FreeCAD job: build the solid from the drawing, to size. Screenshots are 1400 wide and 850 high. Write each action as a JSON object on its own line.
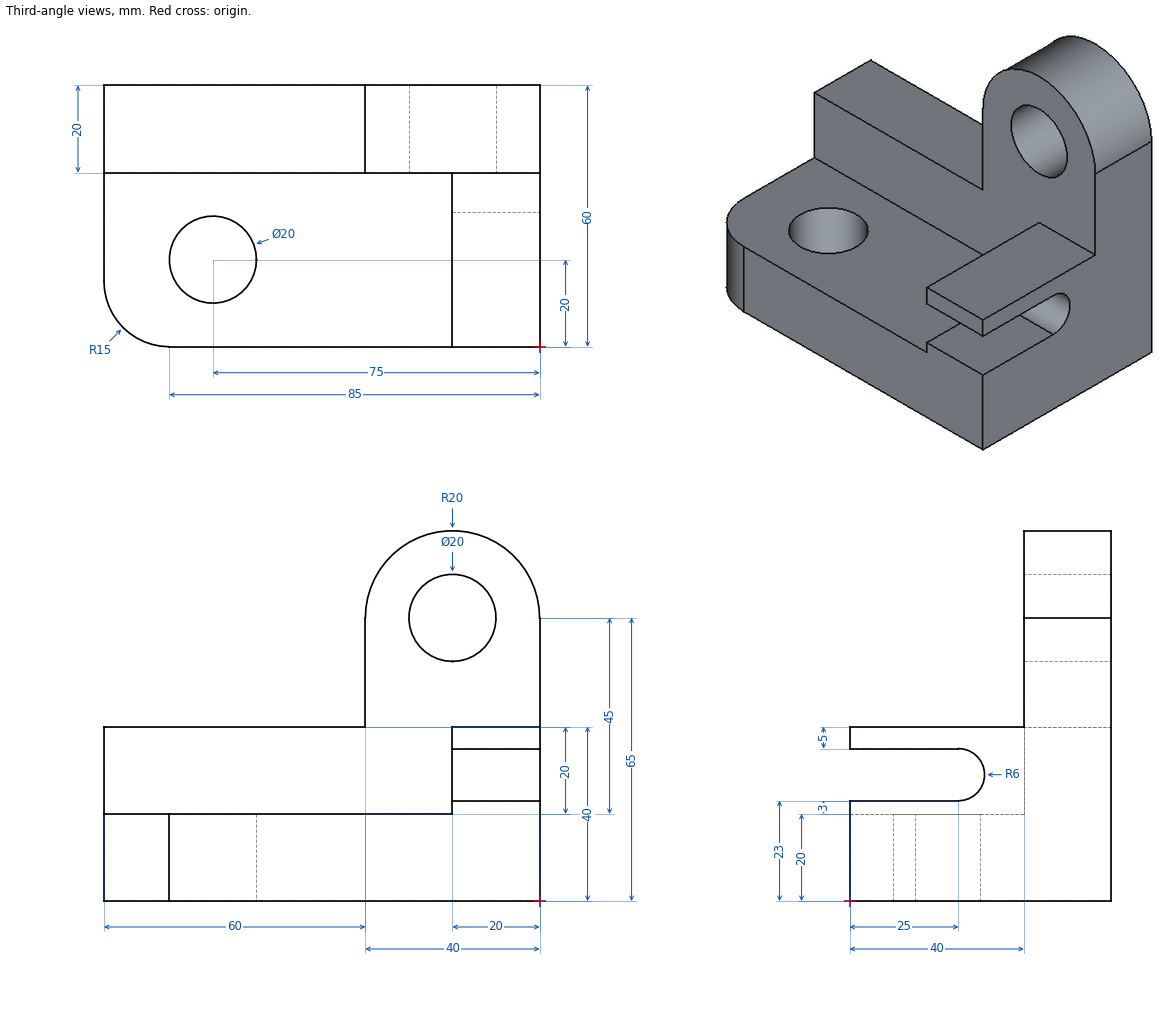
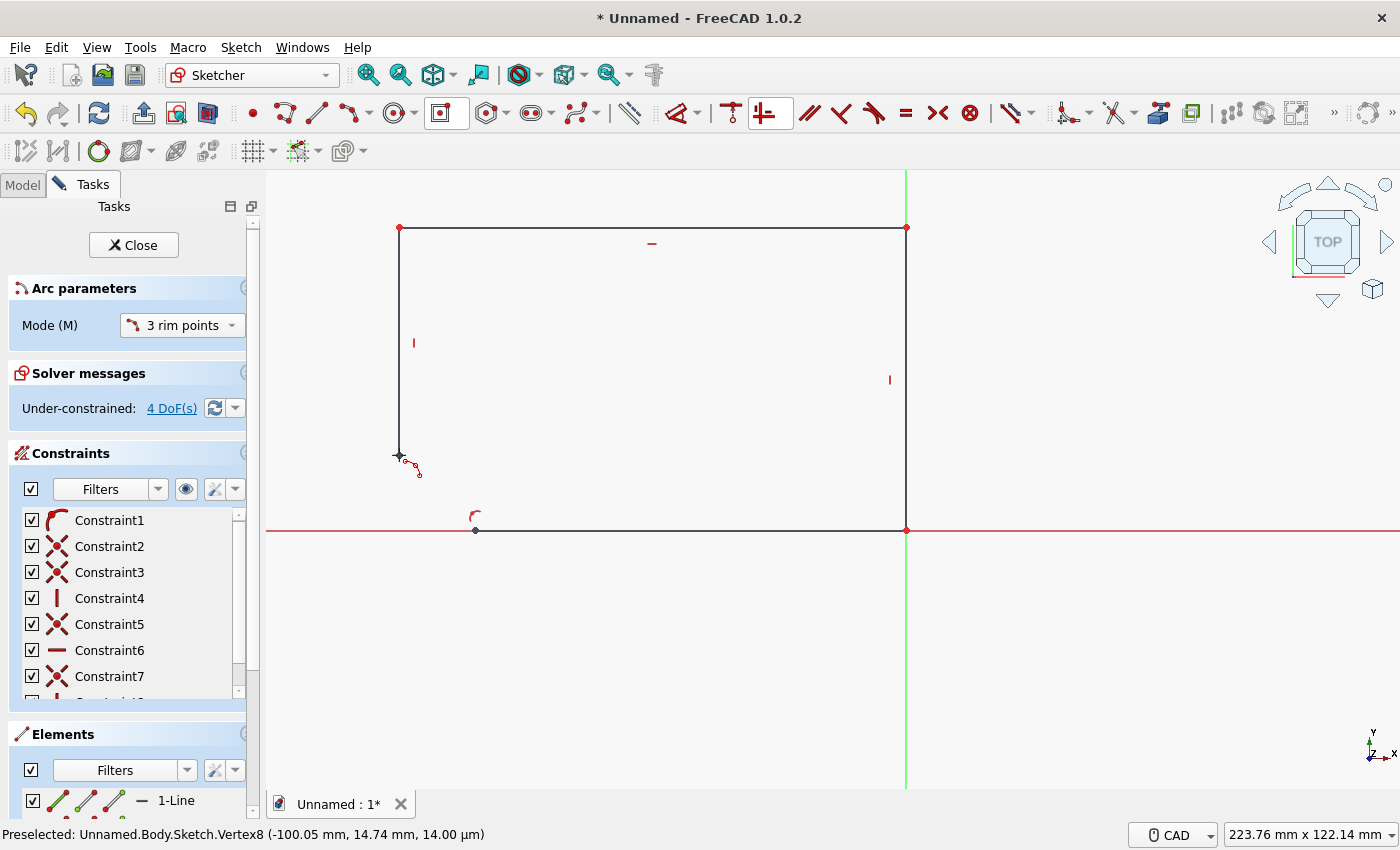
{"action": "left_click", "coordinate": [399, 456]}
{"action": "left_click", "coordinate": [475, 531]}
{"action": "left_click", "coordinate": [421, 508]}
{"action": "key", "text": "Escape"}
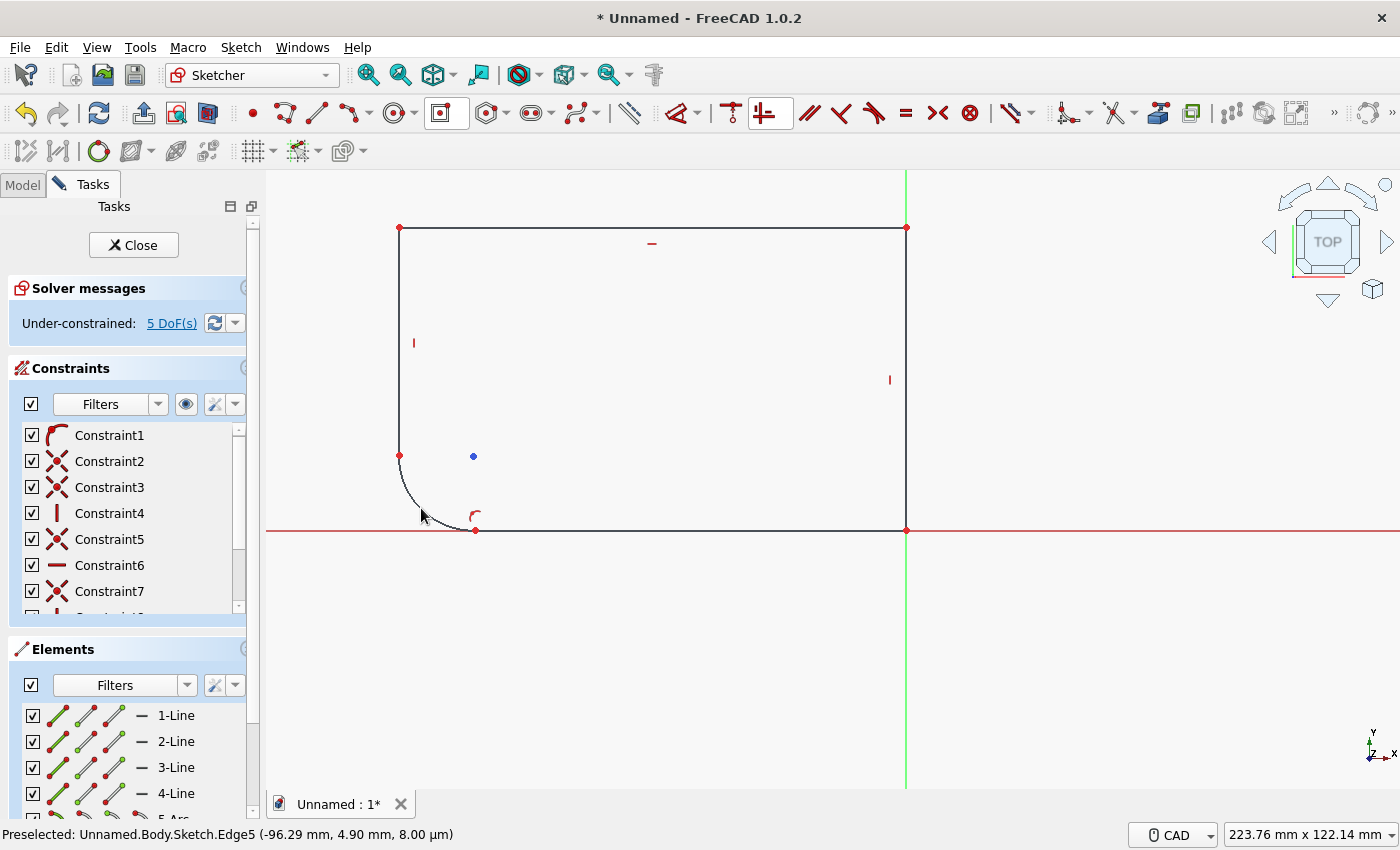
{"action": "left_click", "coordinate": [604, 531]}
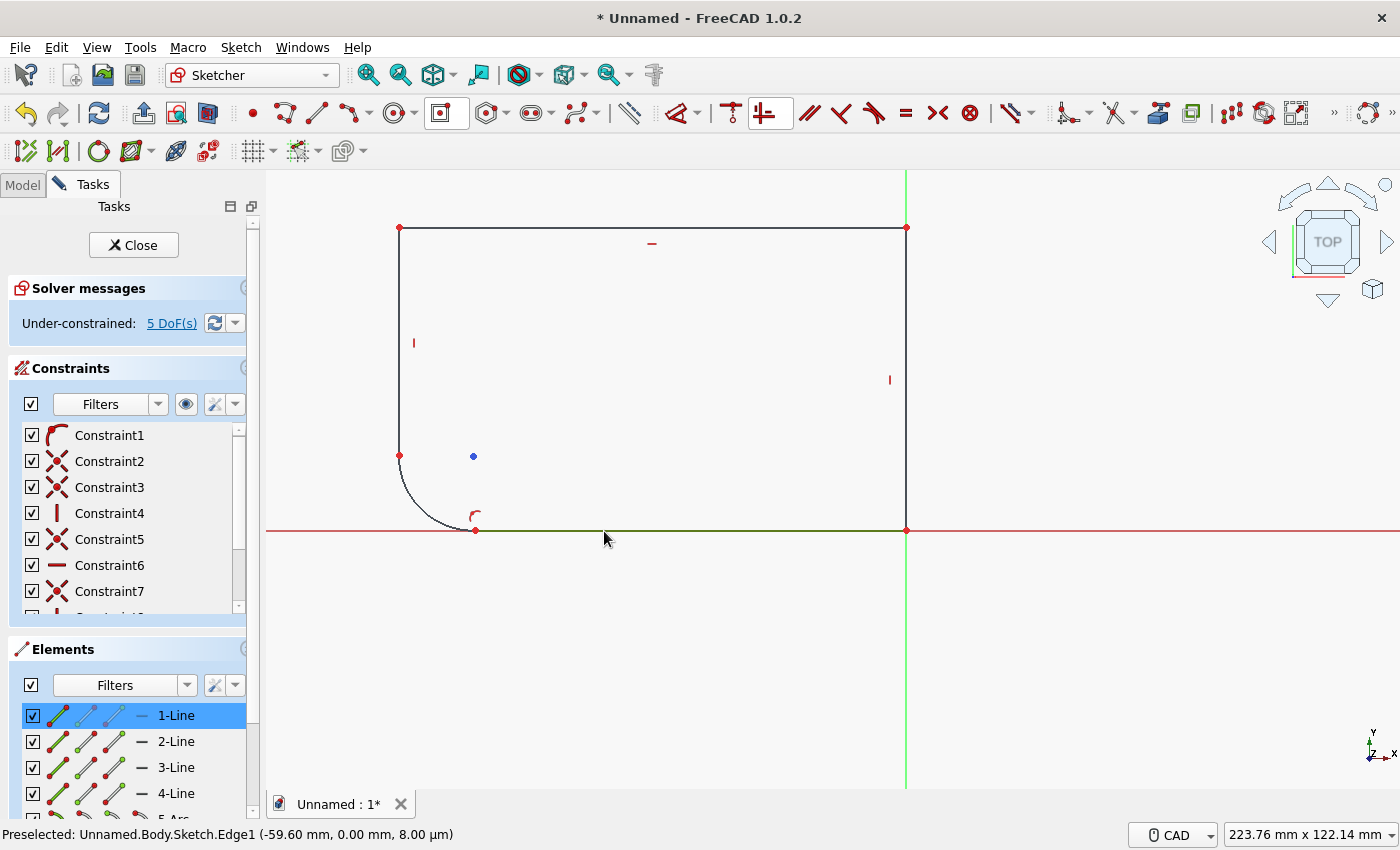
{"action": "left_click", "coordinate": [407, 490]}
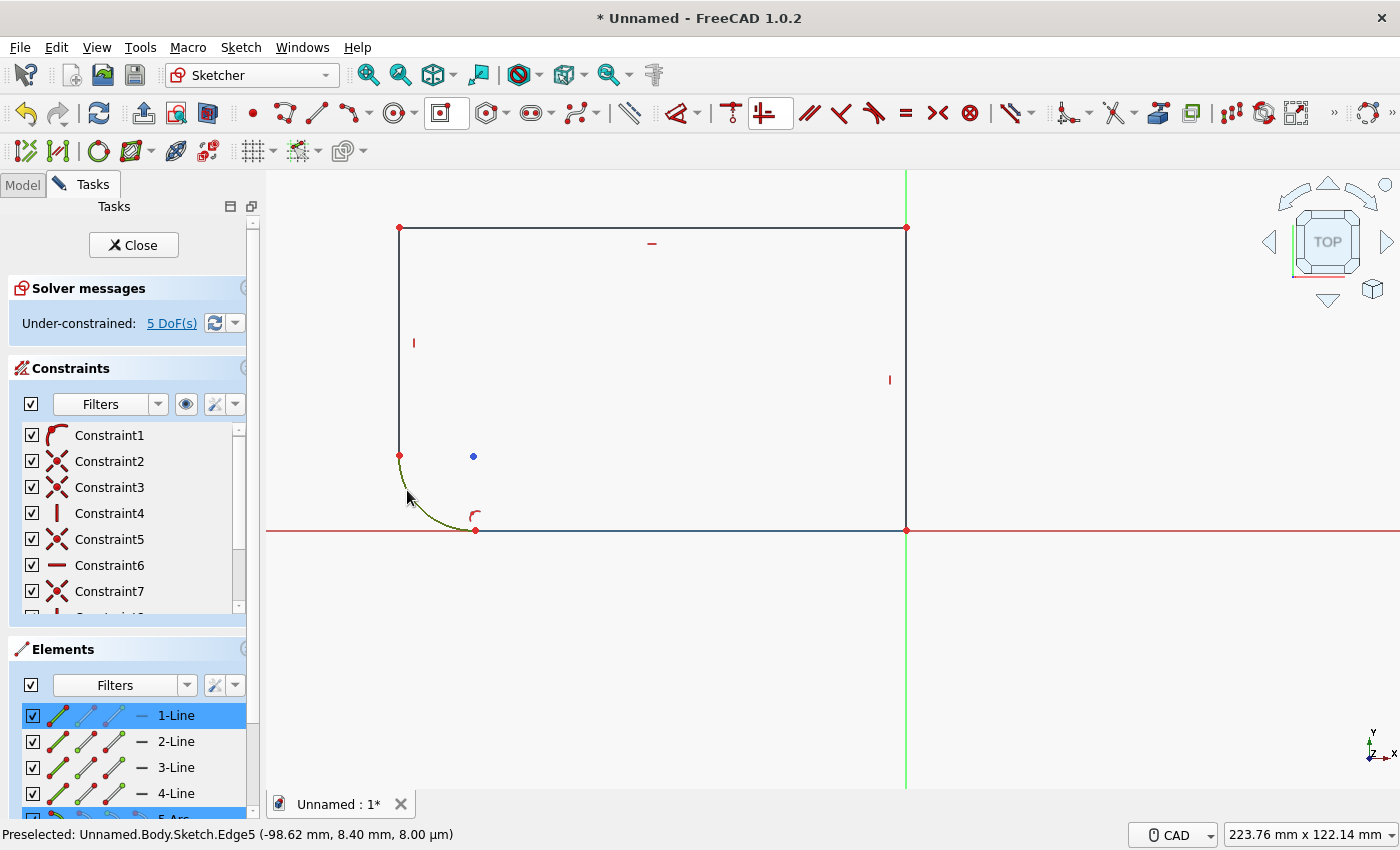
{"action": "left_click", "coordinate": [874, 114]}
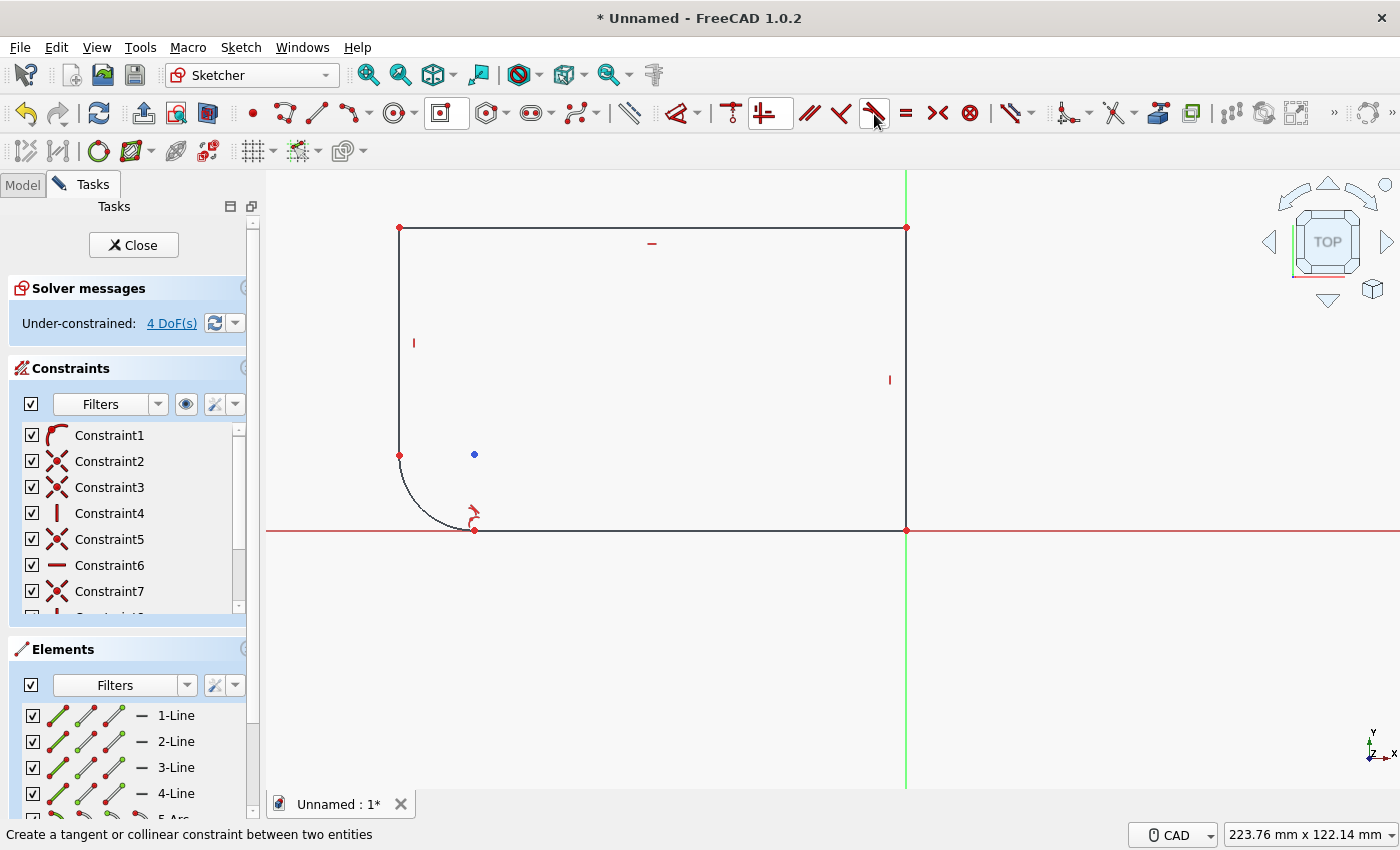
{"action": "left_click", "coordinate": [399, 296]}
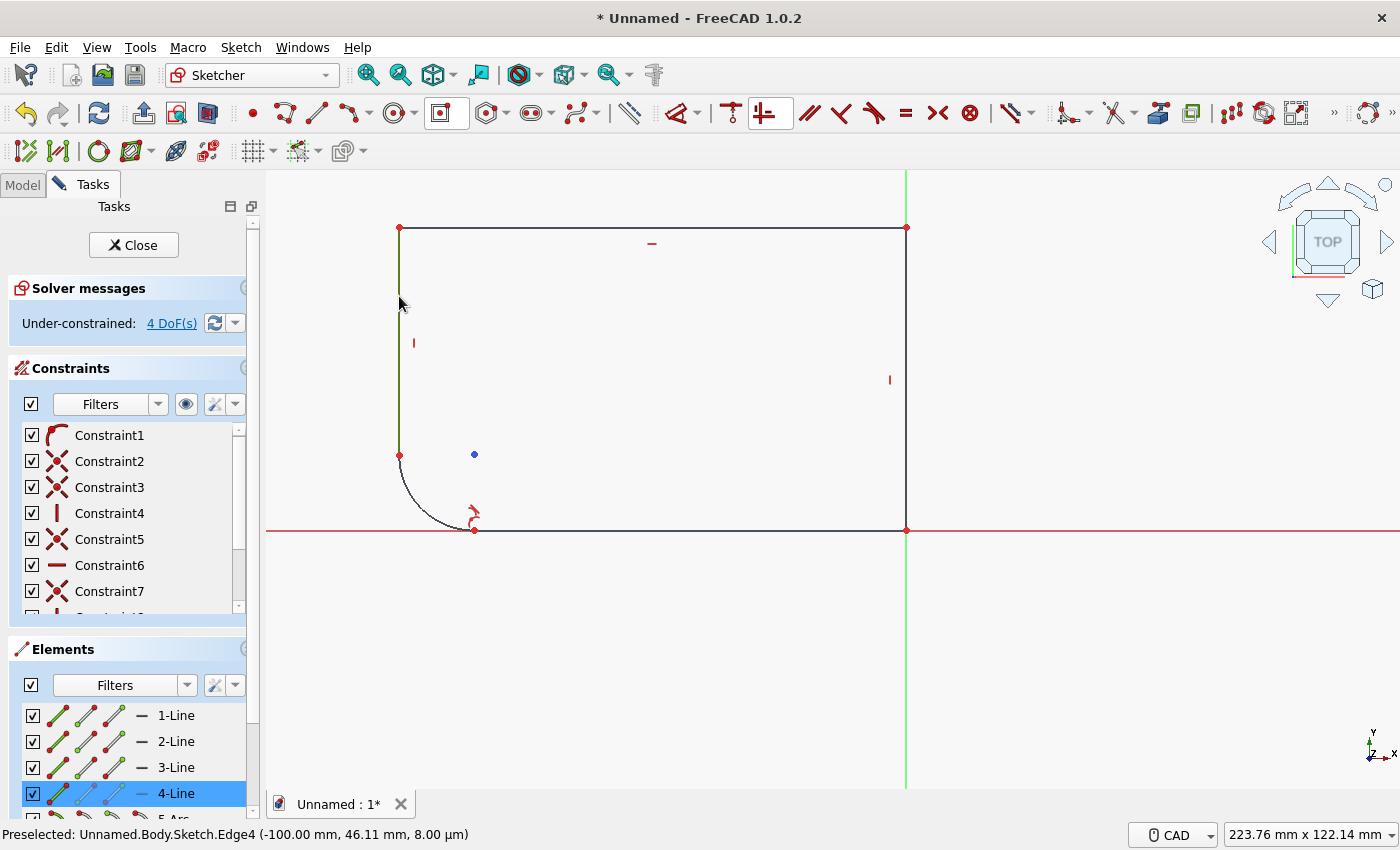
{"action": "left_click", "coordinate": [408, 490]}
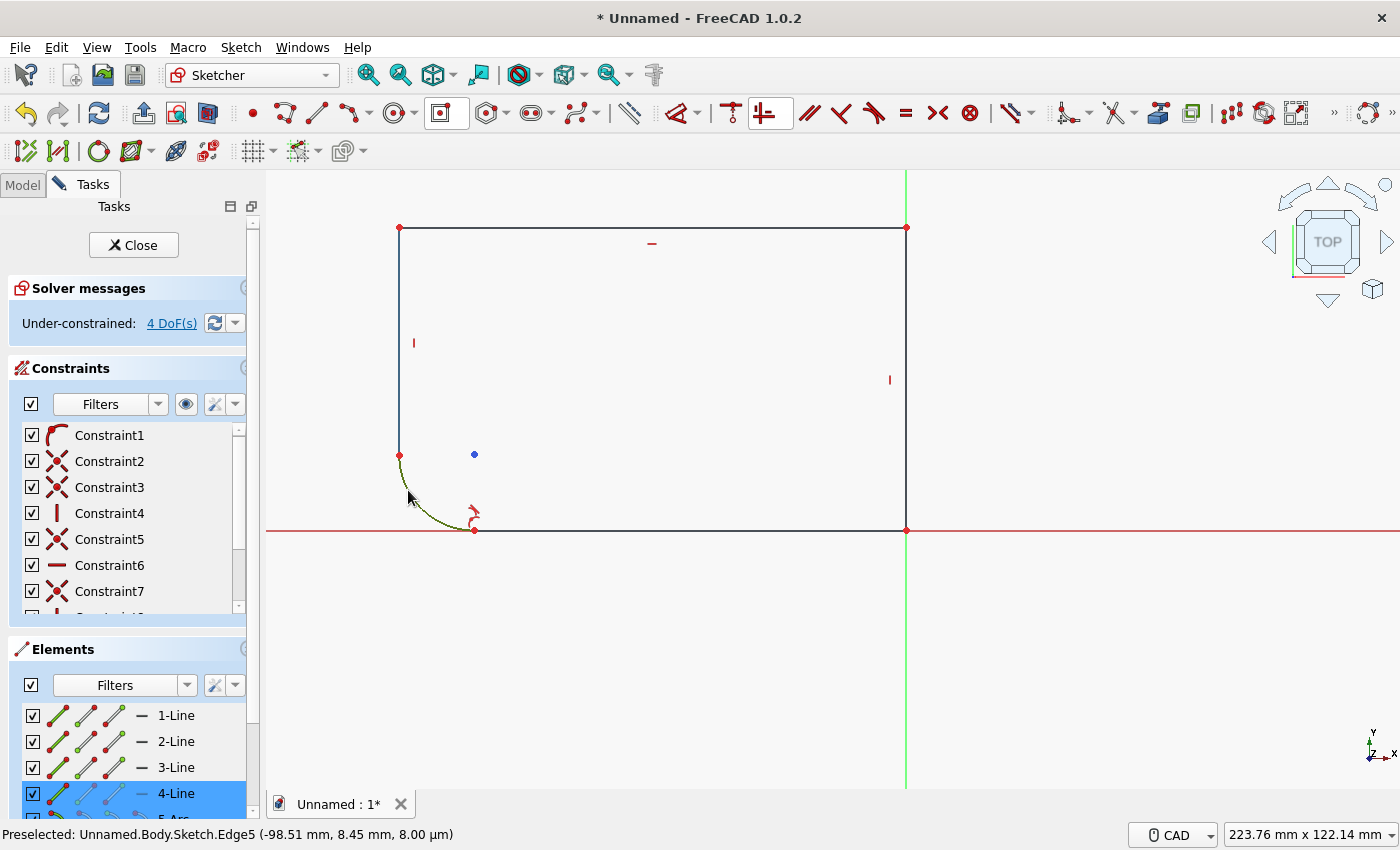
{"action": "key", "text": "t"}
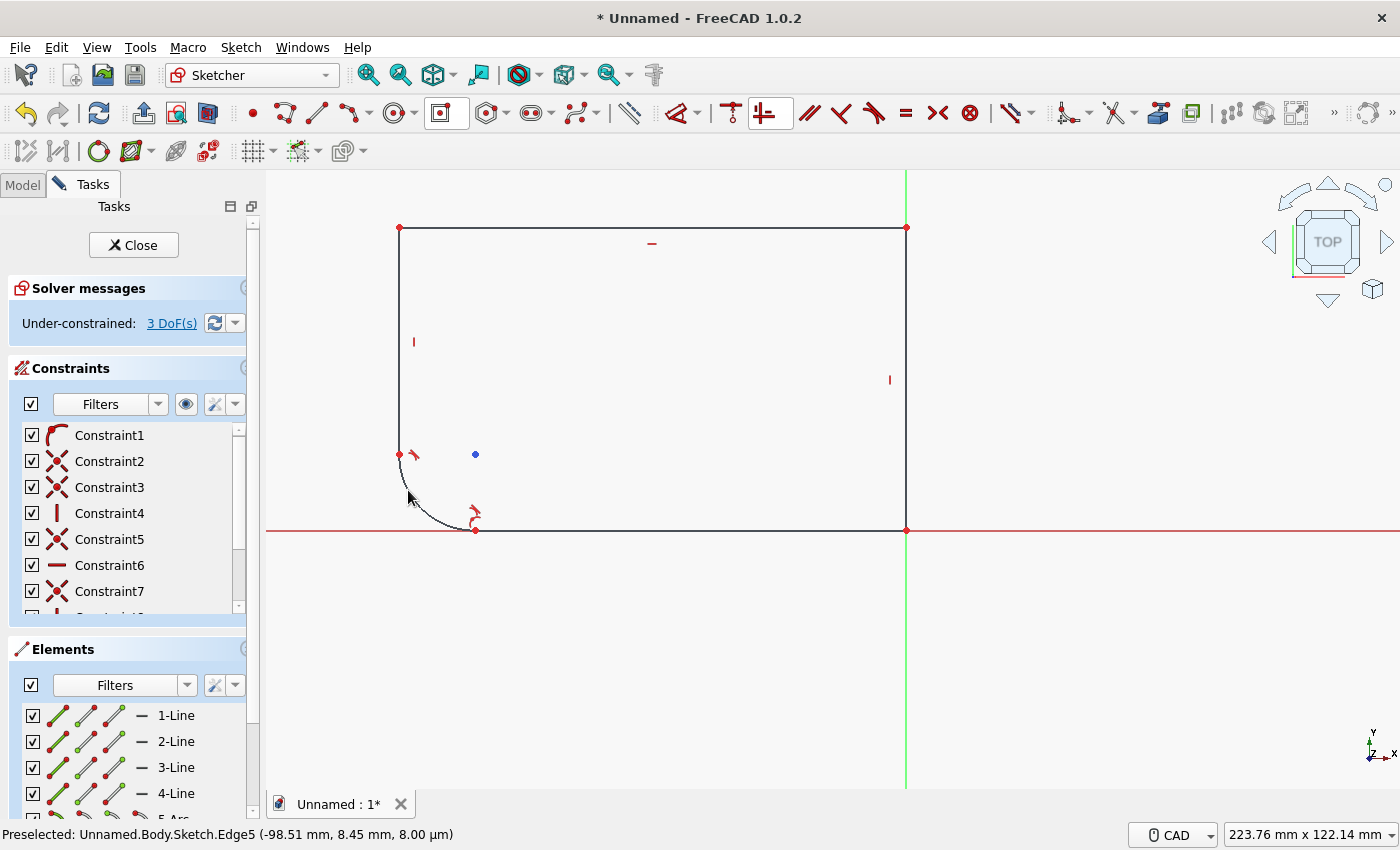
{"action": "left_click", "coordinate": [676, 114]}